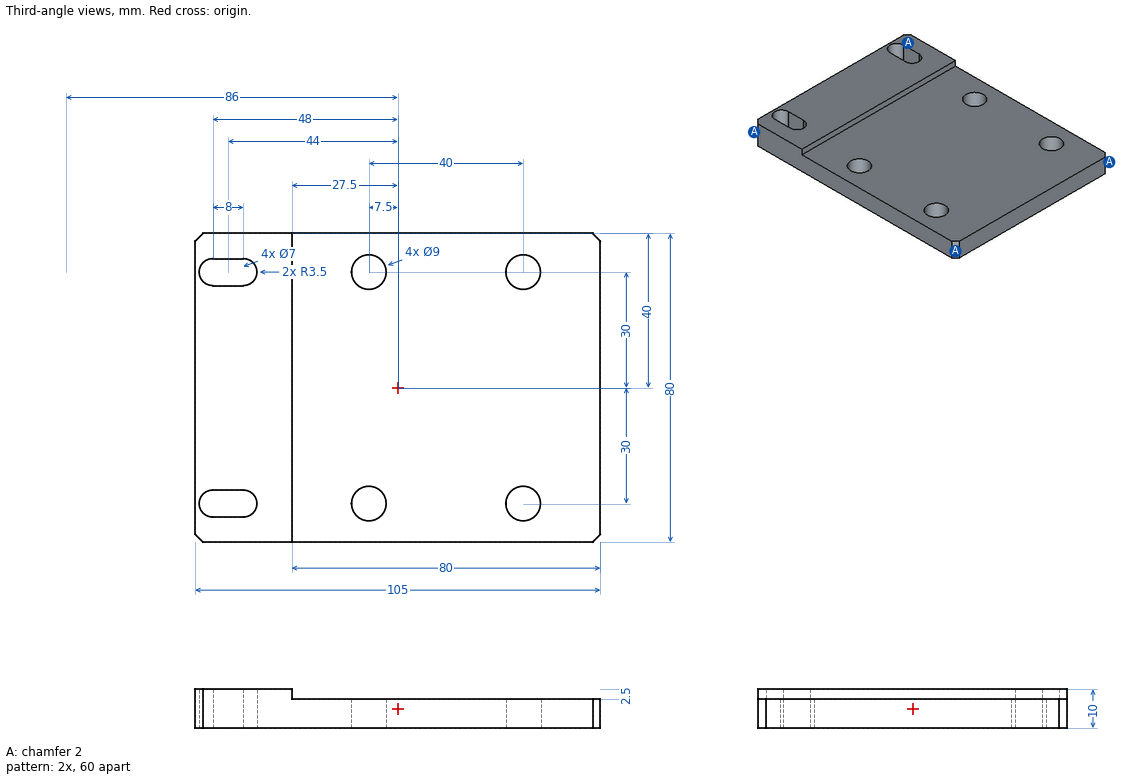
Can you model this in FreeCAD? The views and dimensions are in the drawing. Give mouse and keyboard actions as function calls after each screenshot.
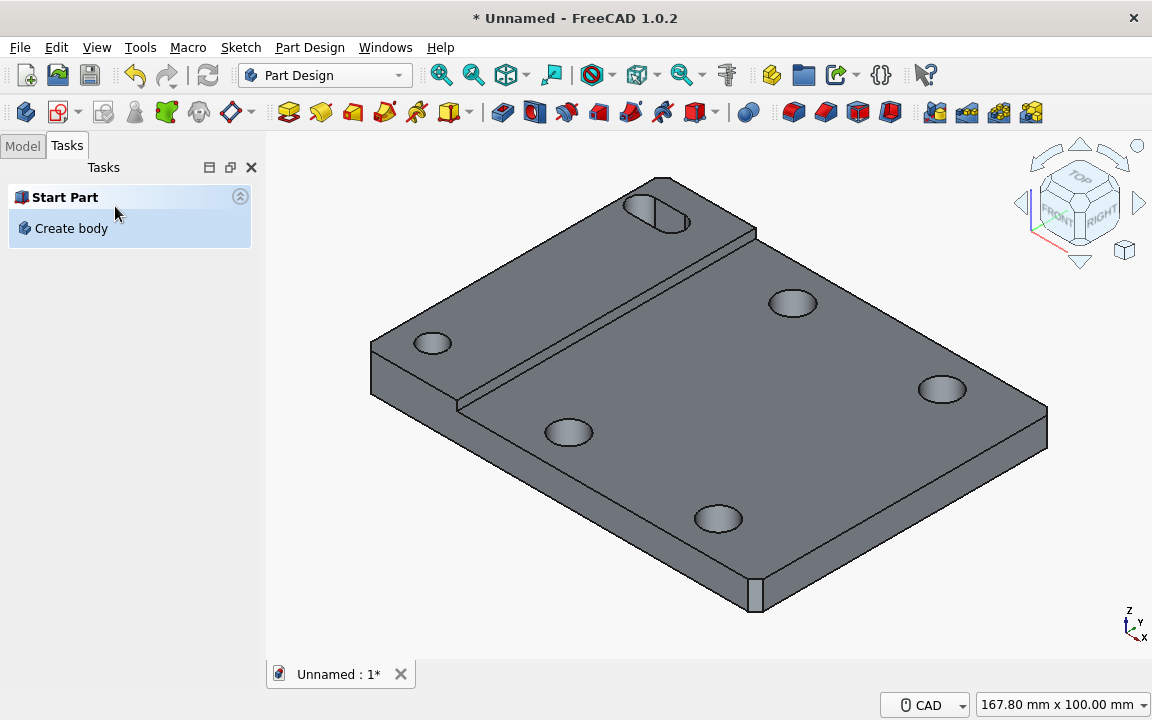
click(23, 145)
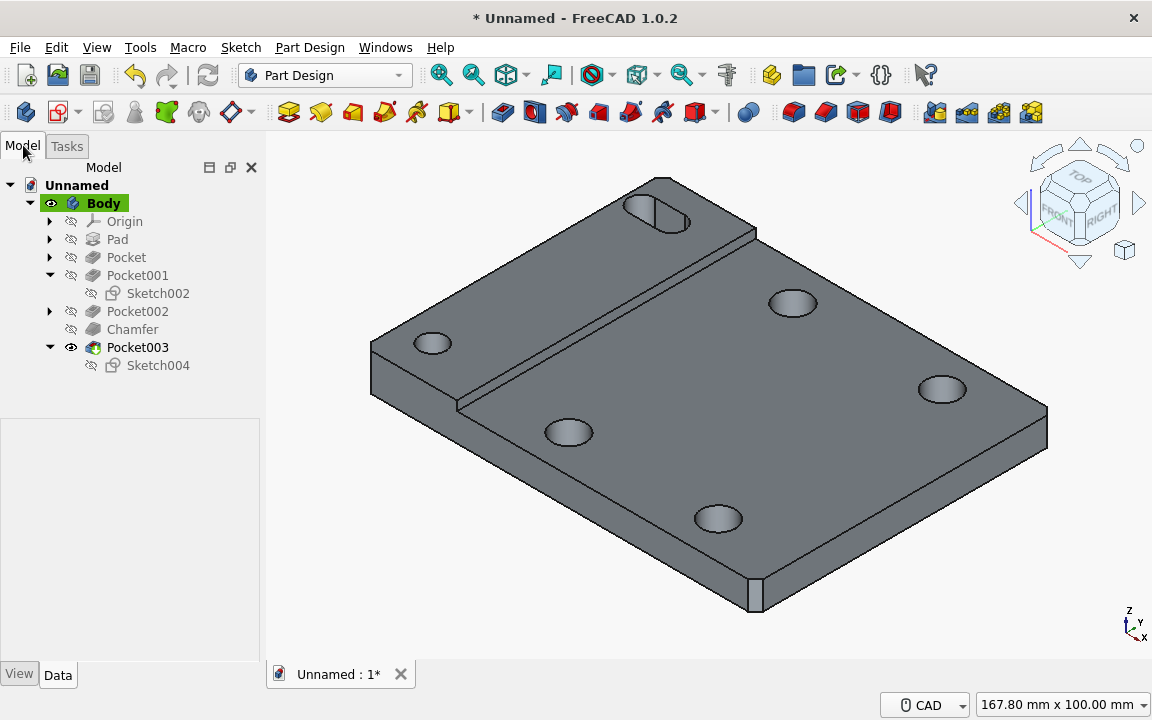
click(116, 347)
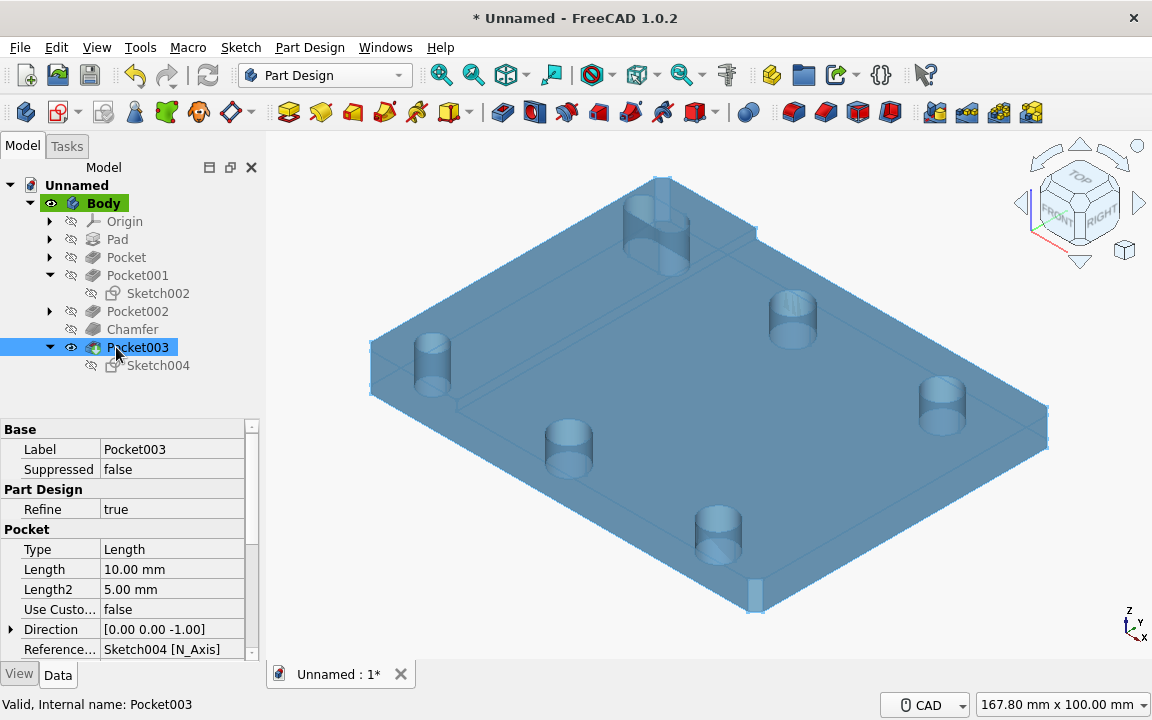
click(968, 112)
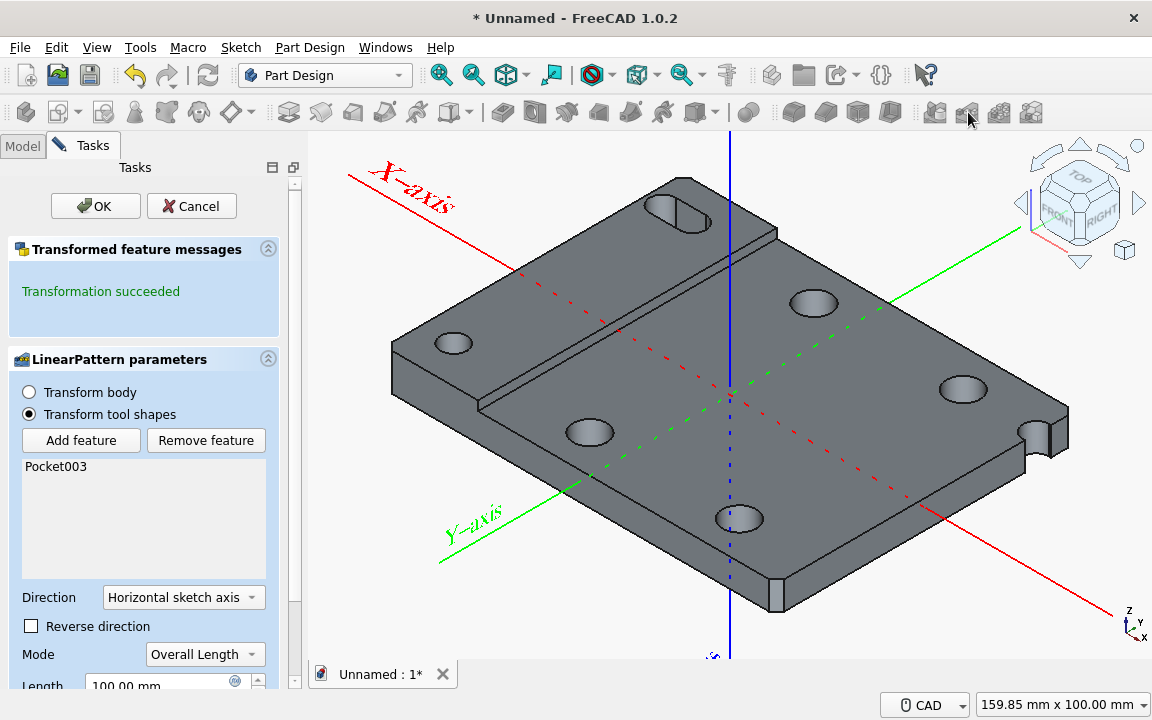
click(184, 598)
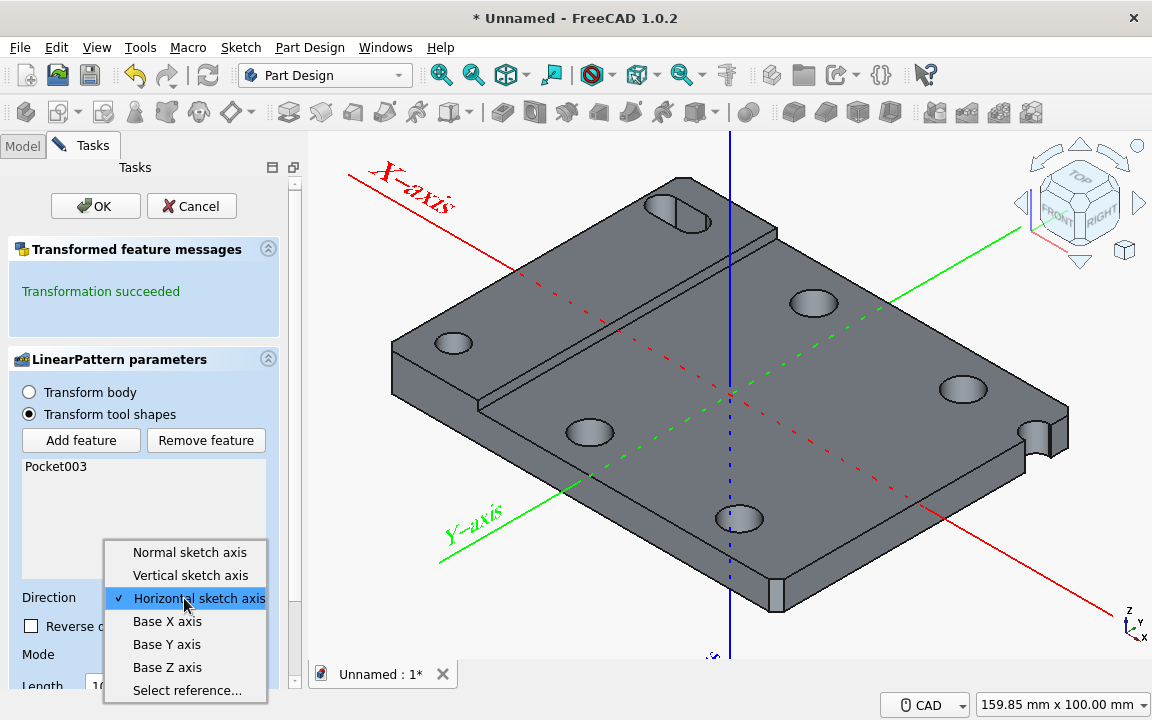
click(184, 644)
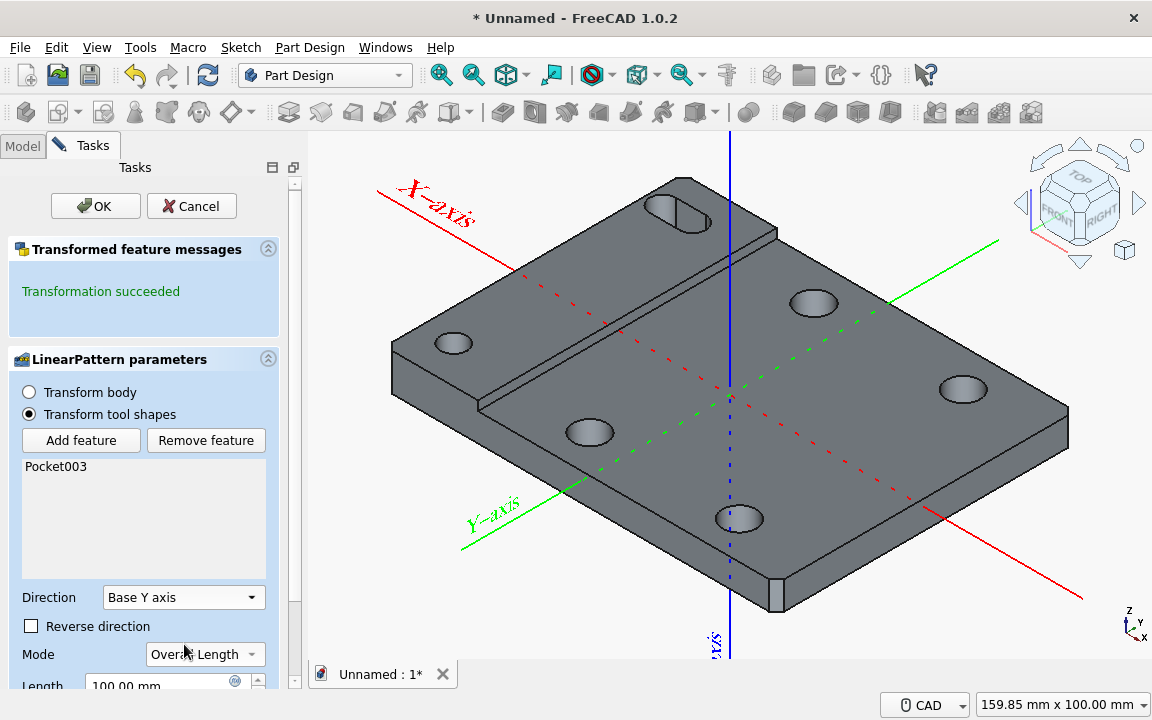
click(206, 654)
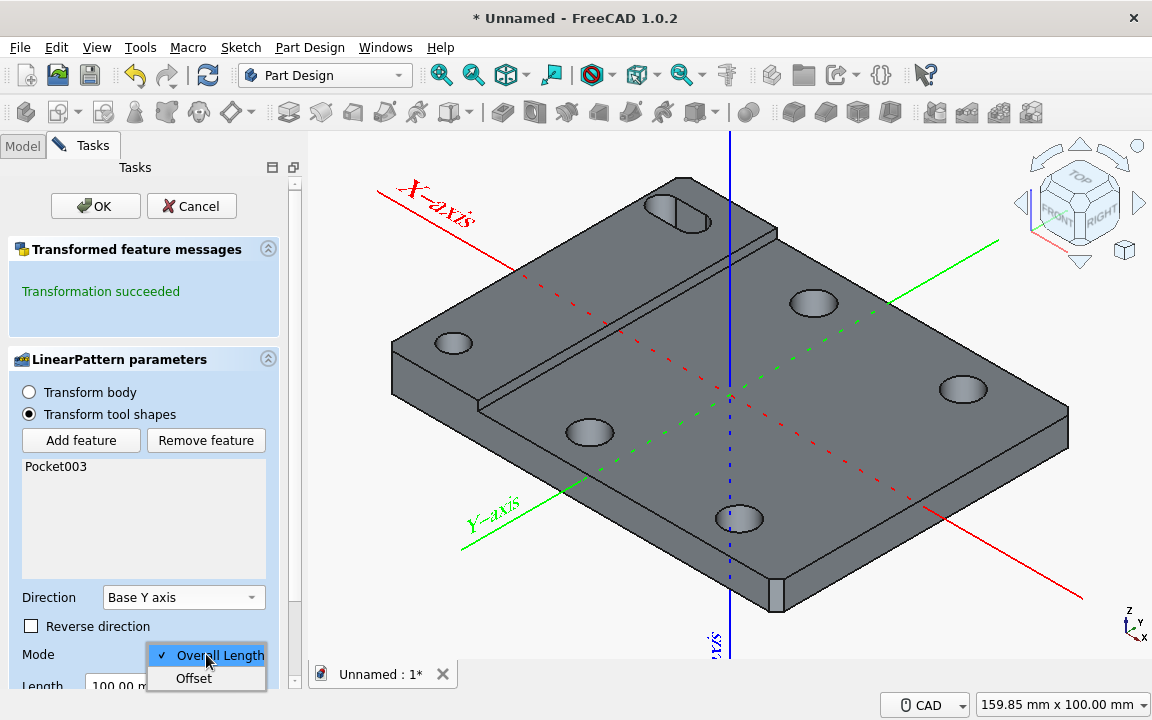
click(206, 678)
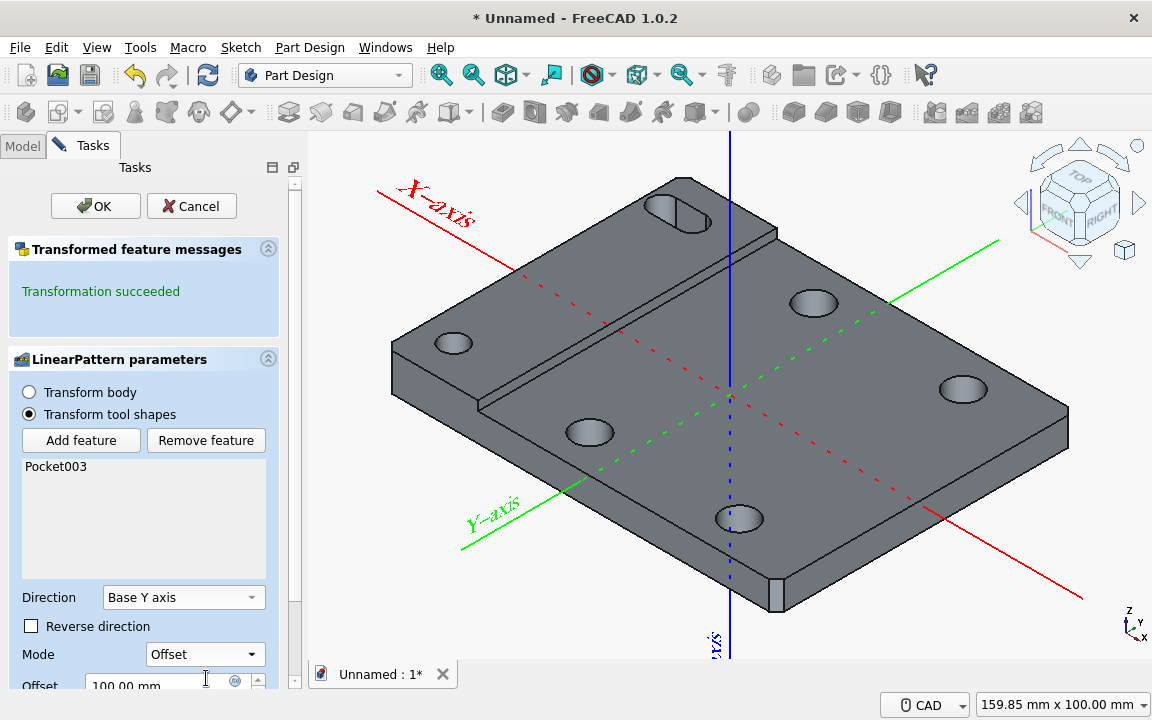
scroll(295, 432, down, 2)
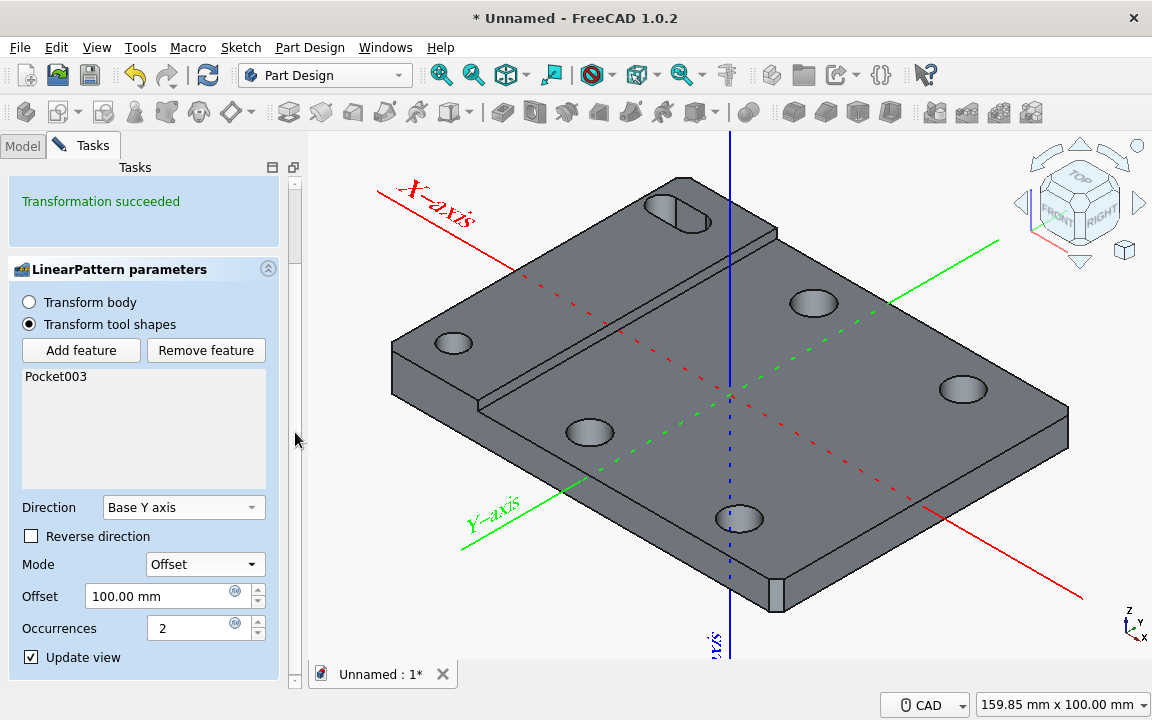
triple_click(168, 596)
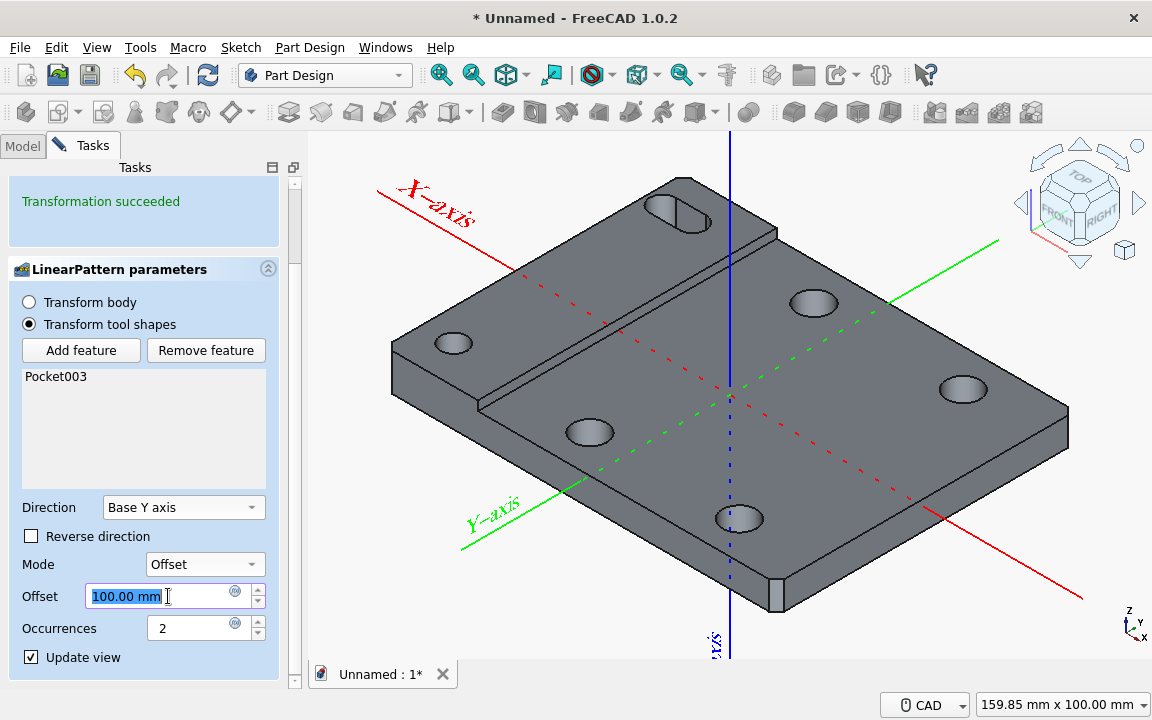
text(60)
key(Tab)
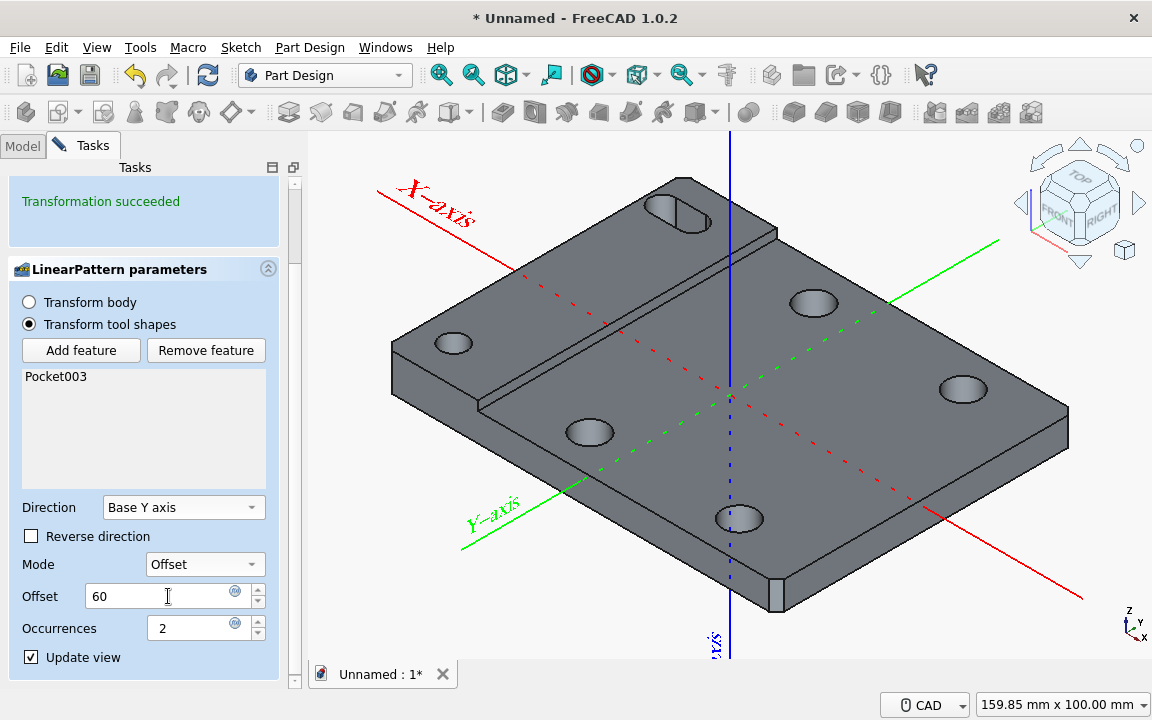
triple_click(198, 628)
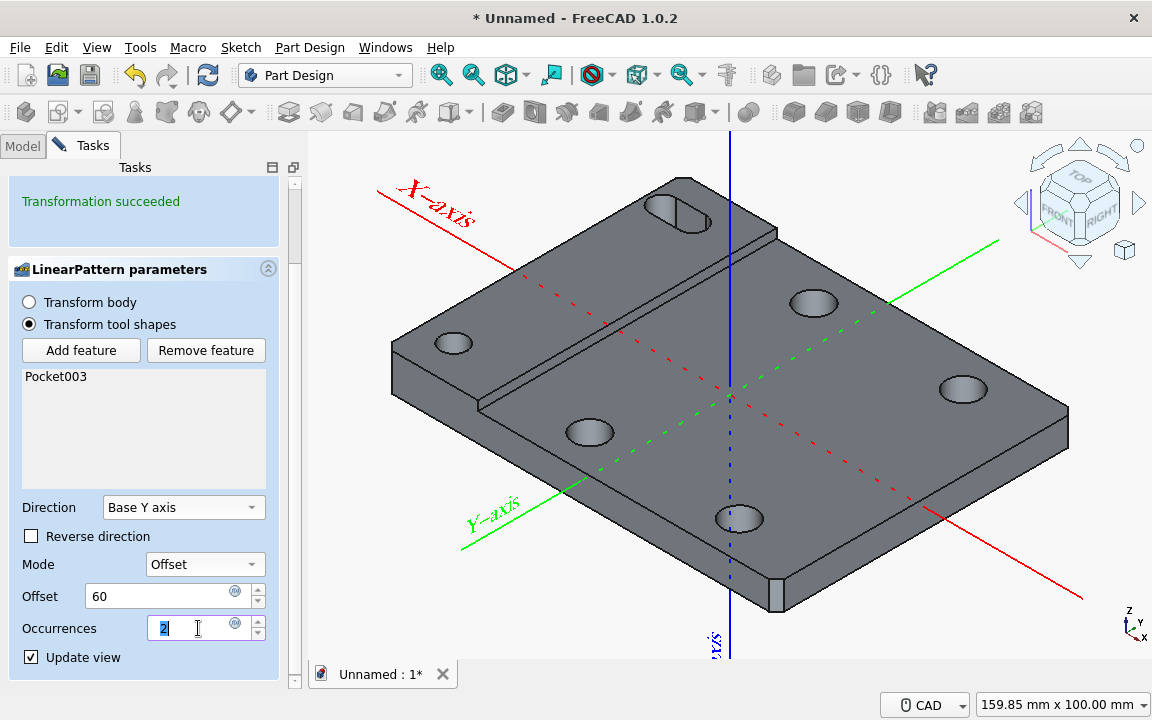
text(2)
key(Tab)